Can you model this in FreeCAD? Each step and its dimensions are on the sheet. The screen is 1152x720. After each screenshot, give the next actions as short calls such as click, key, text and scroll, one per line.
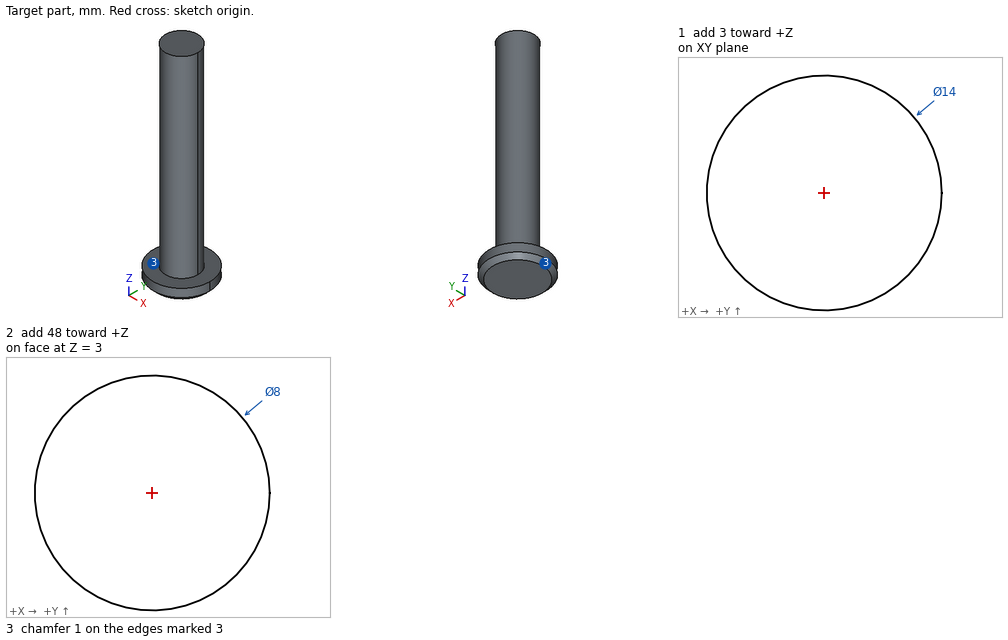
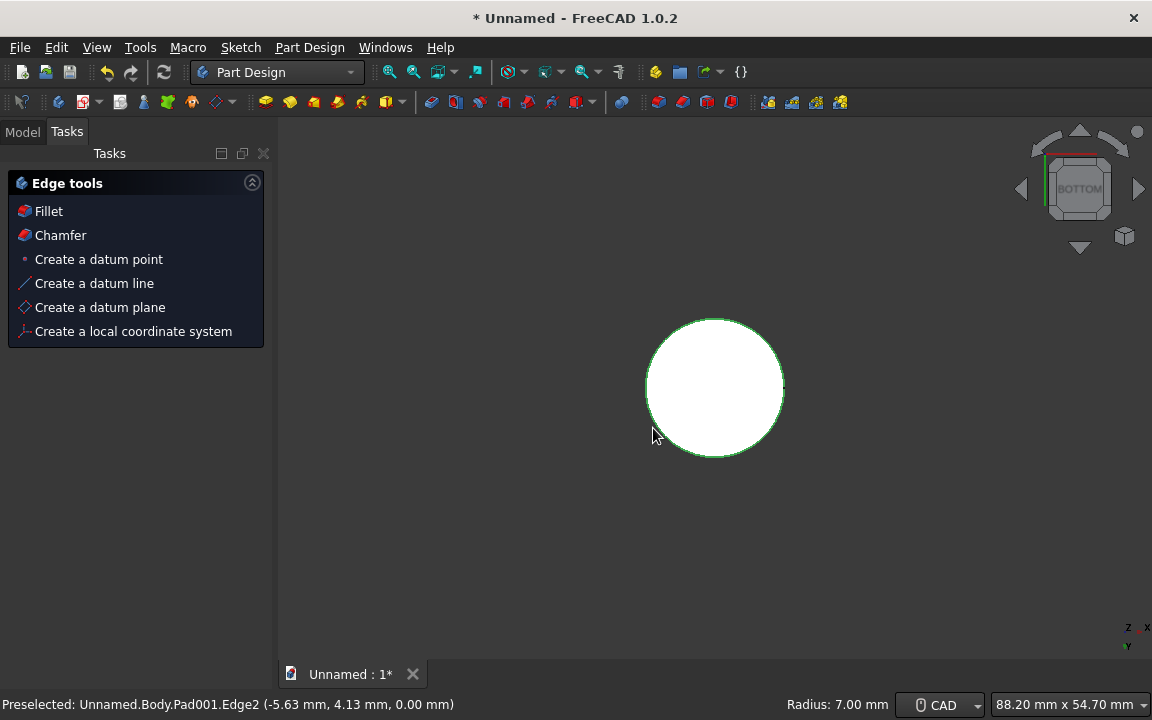
click(684, 102)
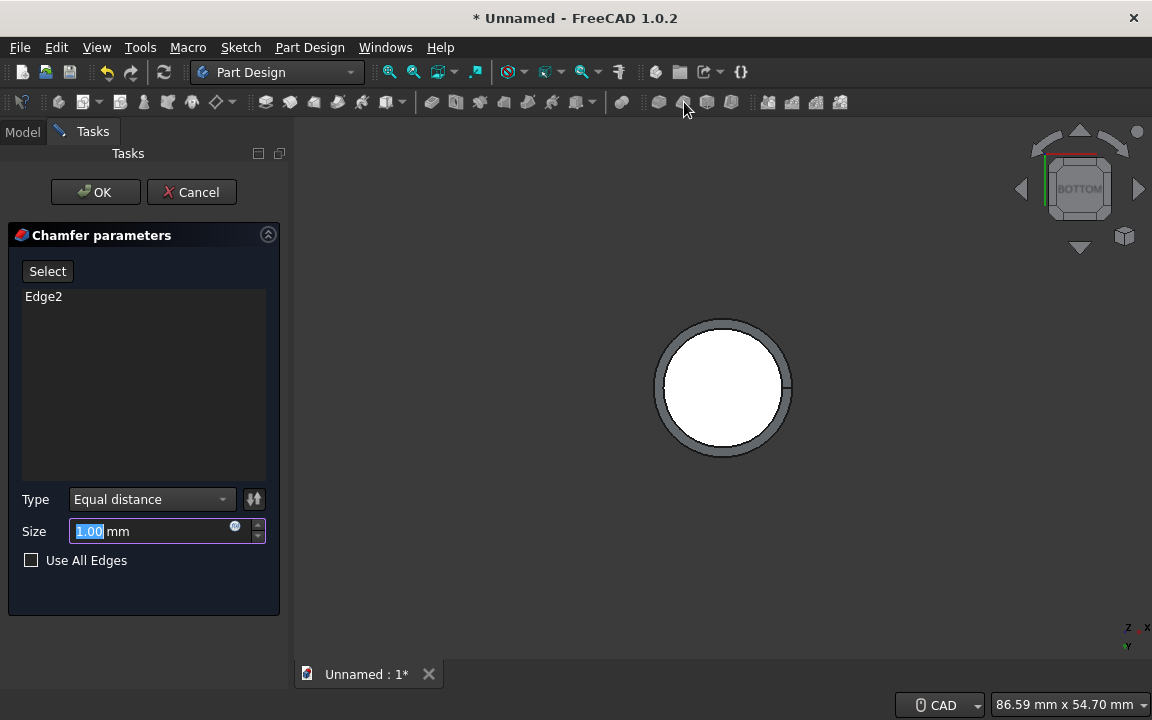
text(1)
key(Tab)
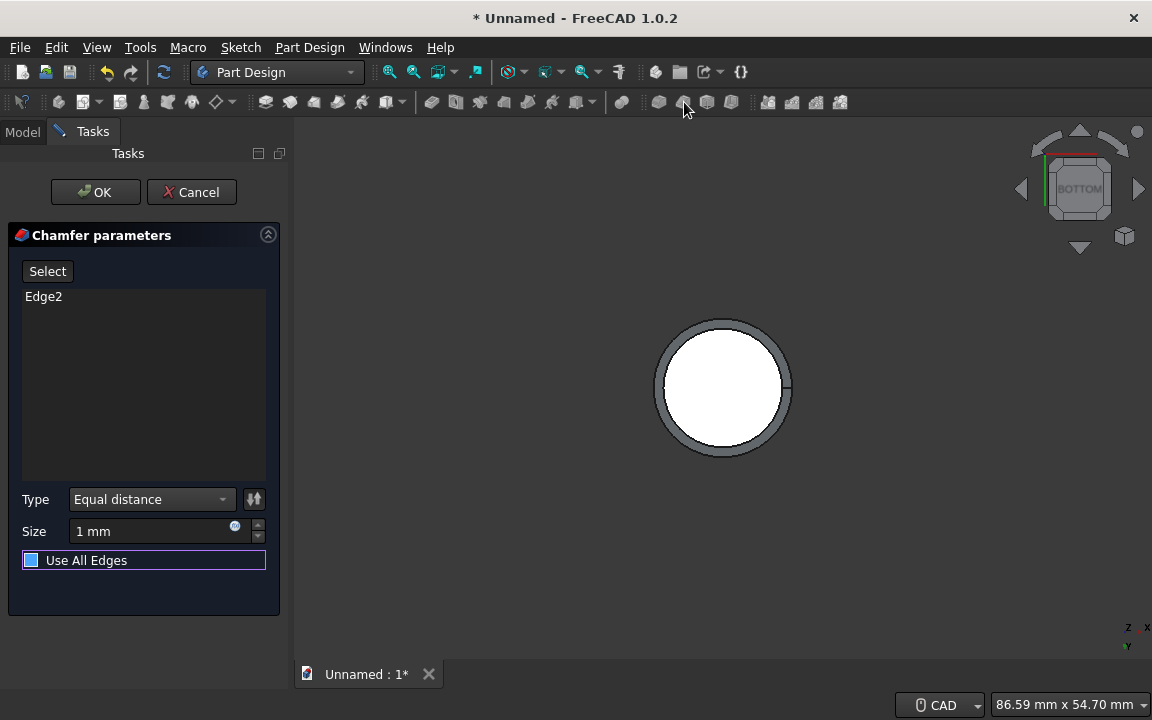
click(96, 192)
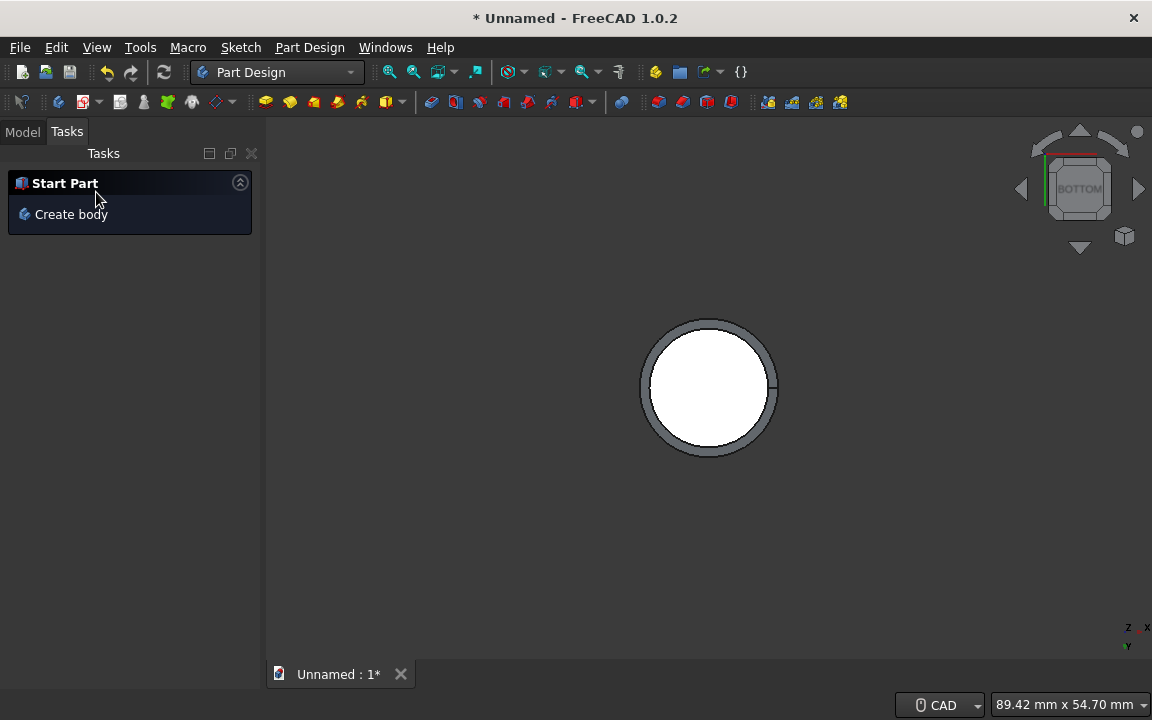
key(0)